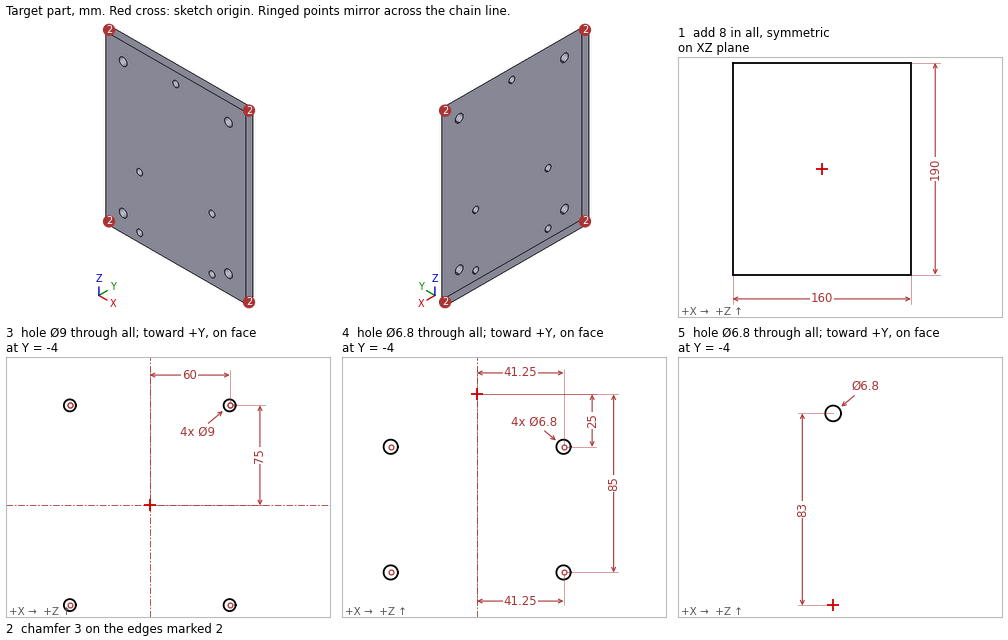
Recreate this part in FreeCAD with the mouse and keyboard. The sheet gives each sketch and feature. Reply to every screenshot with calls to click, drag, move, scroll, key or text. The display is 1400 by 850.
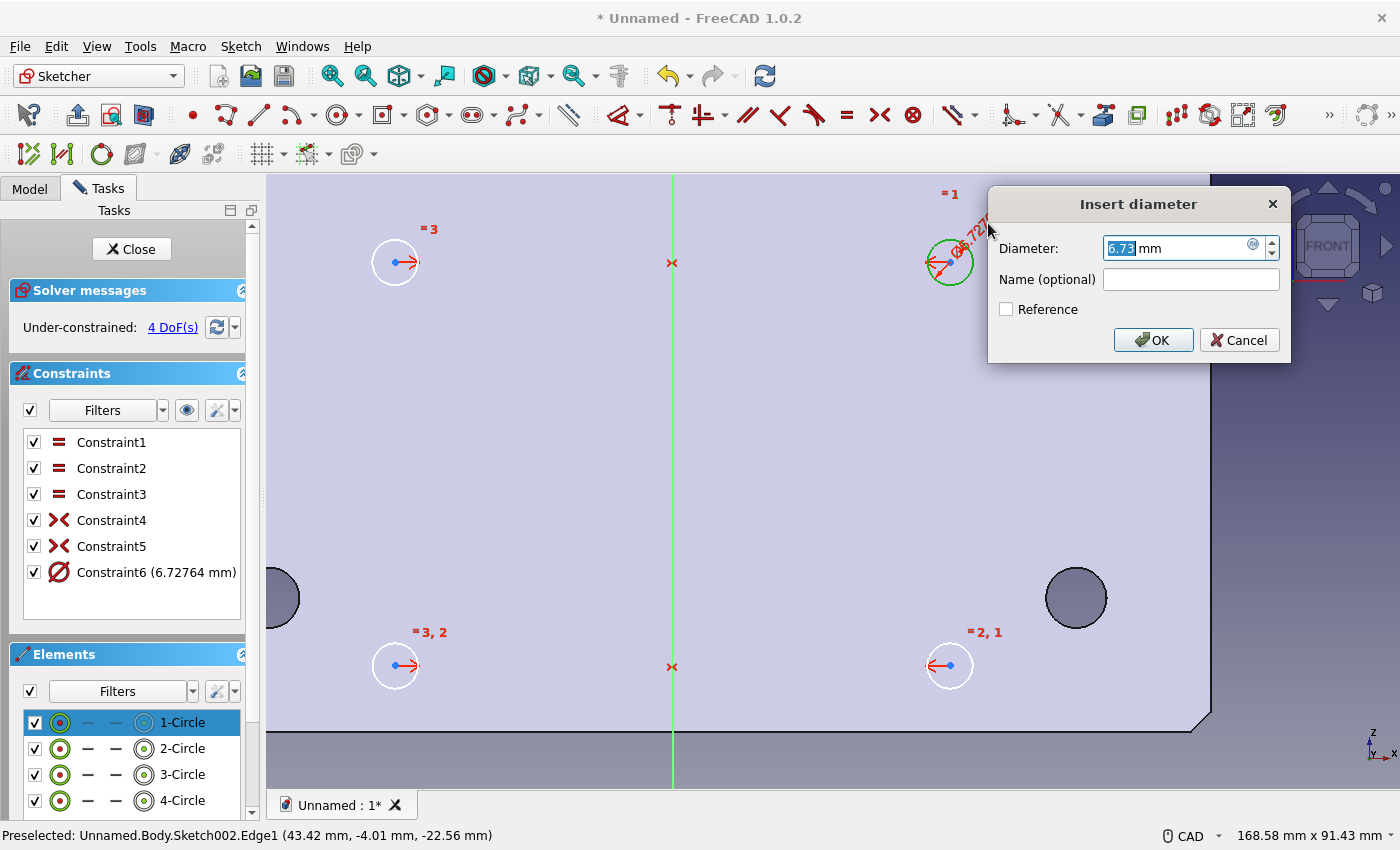
text(6.8)
key(Return)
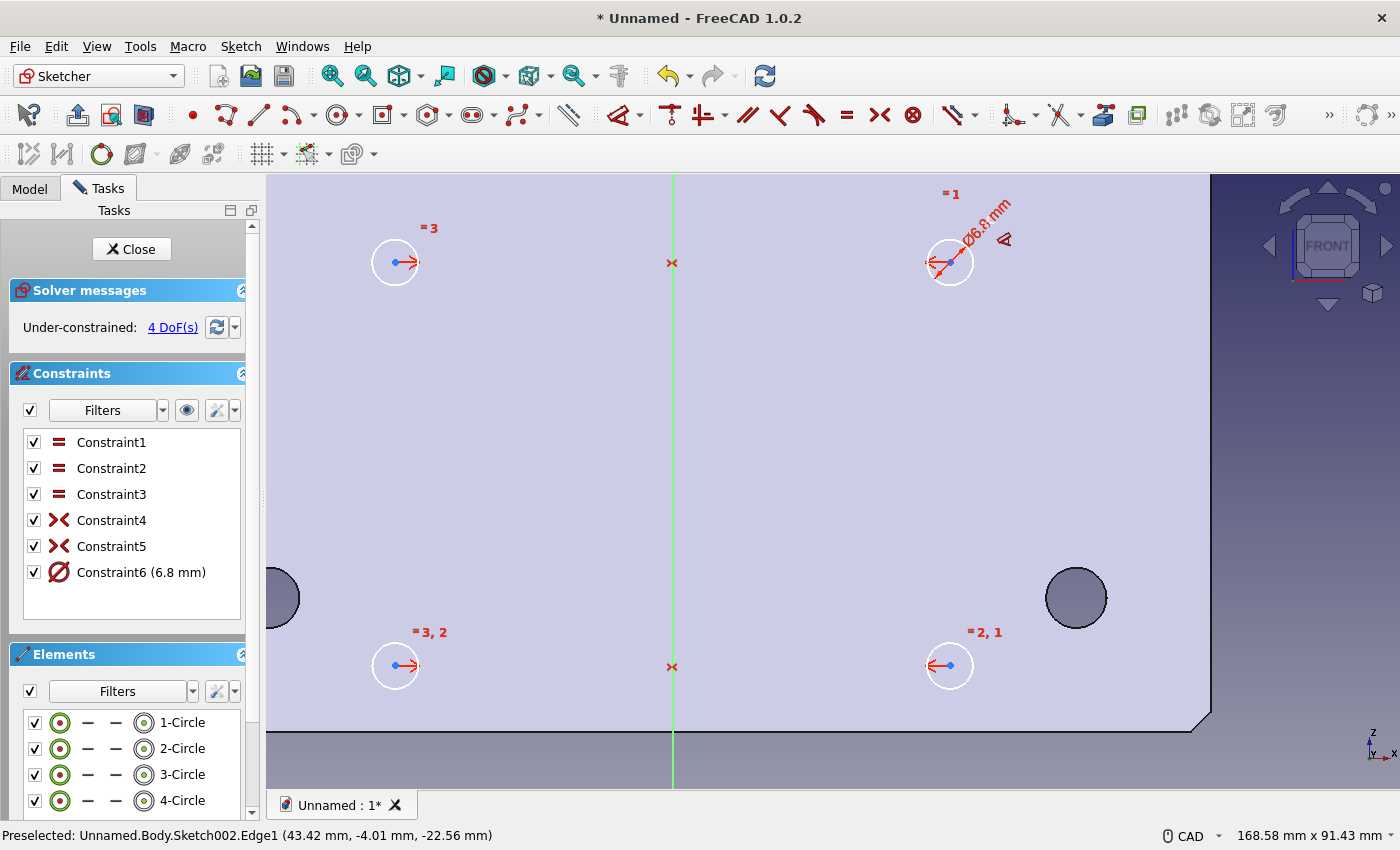
click(950, 262)
click(984, 246)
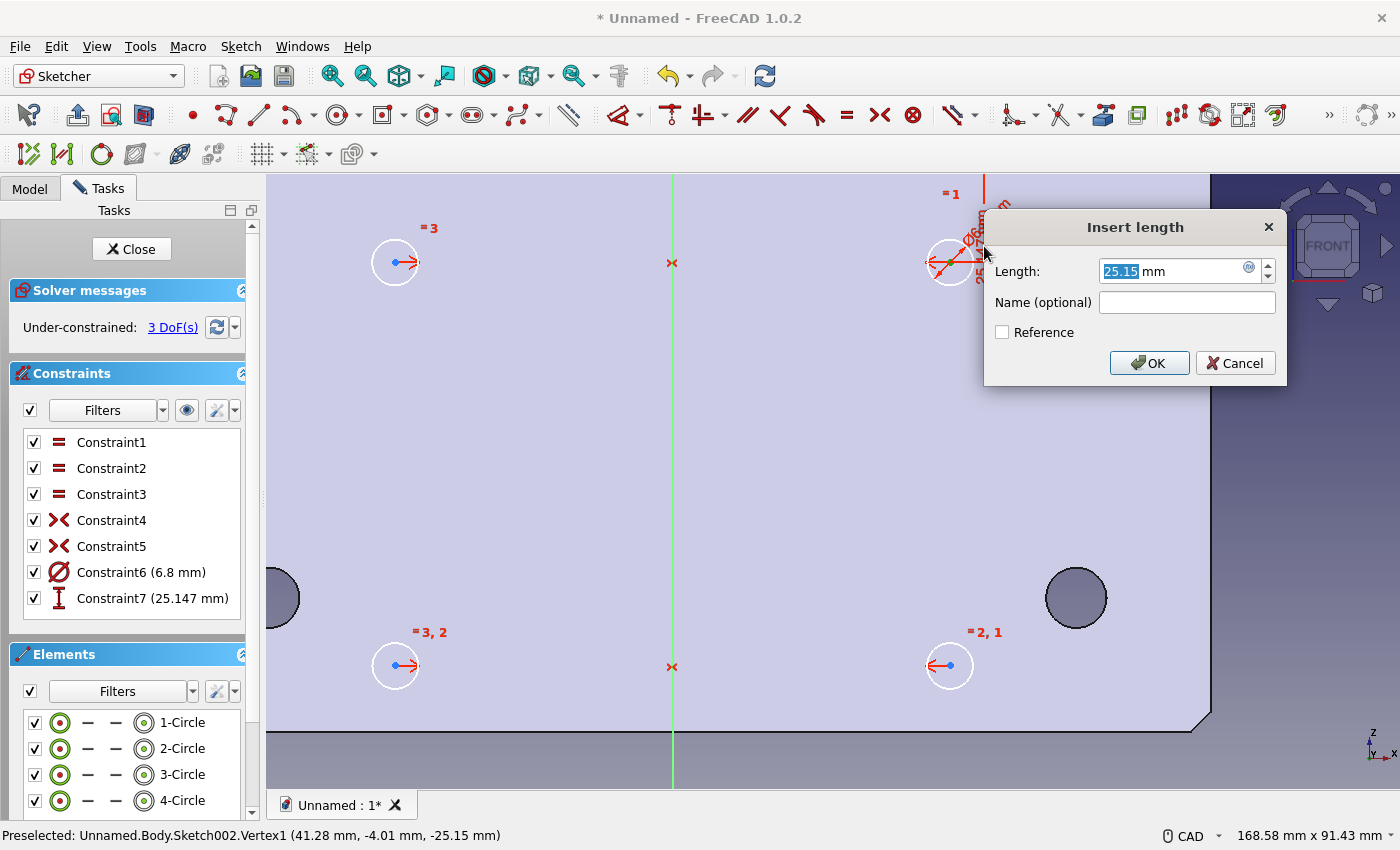
text(25)
key(Return)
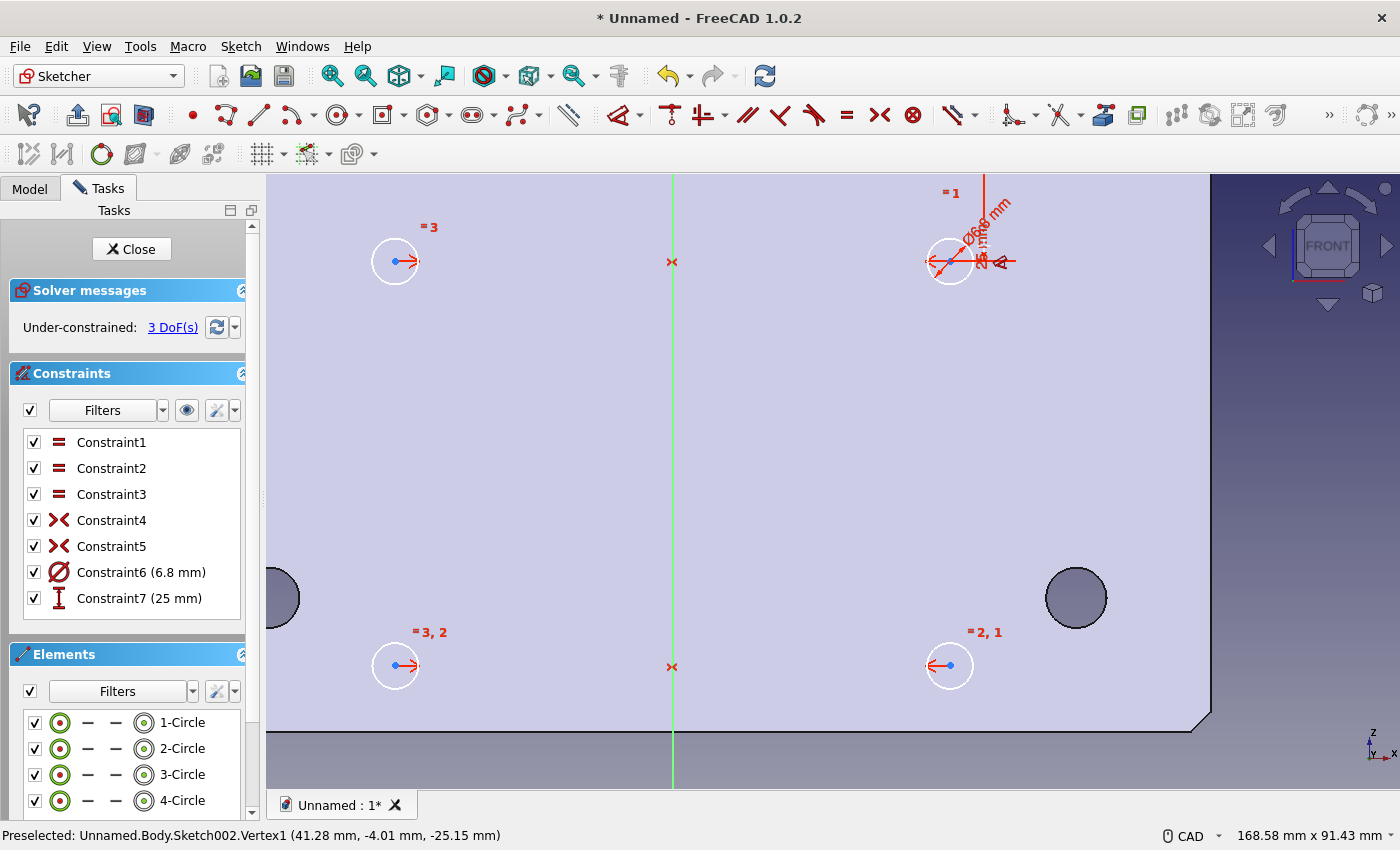
click(950, 666)
click(984, 434)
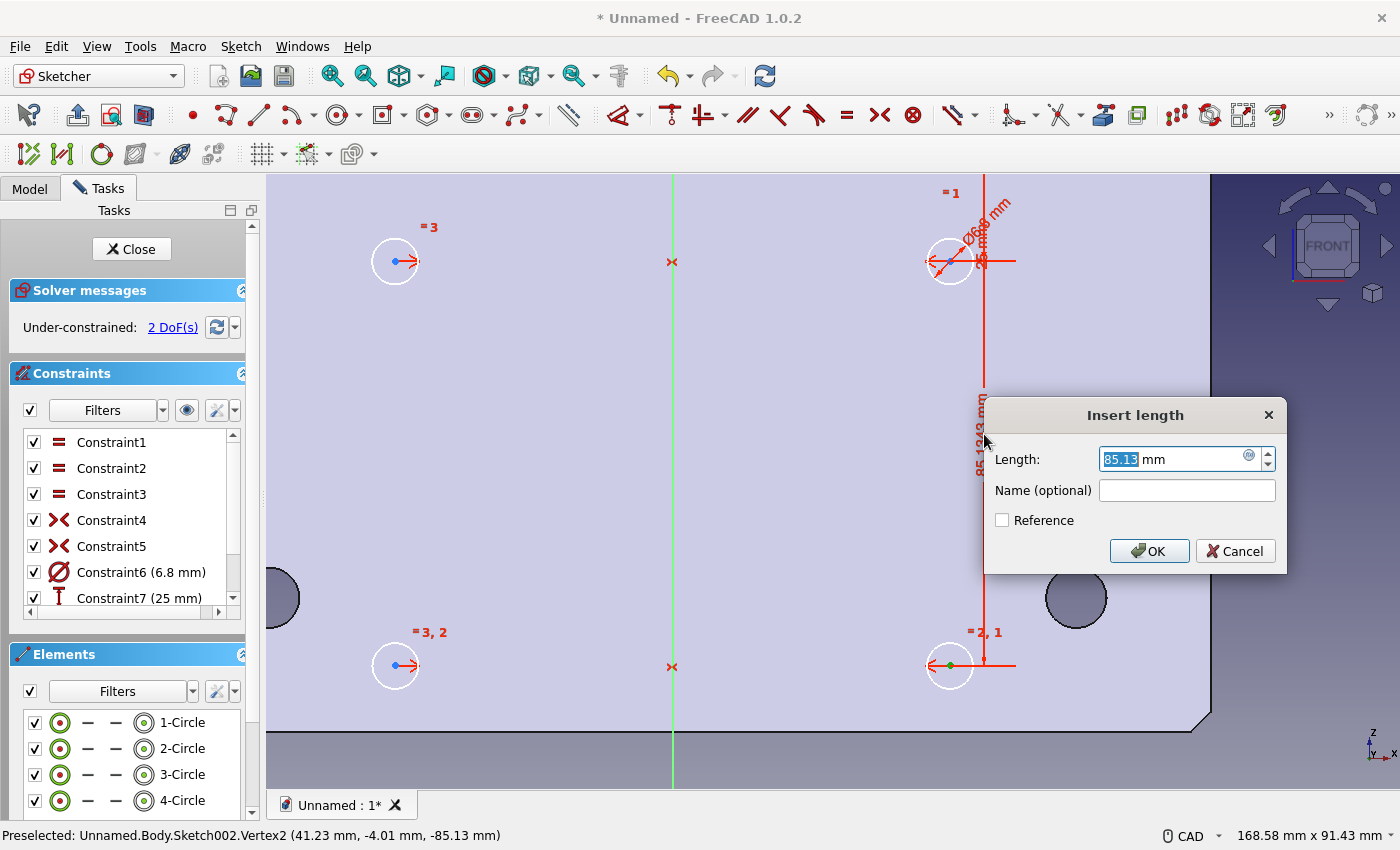
text(85)
key(Return)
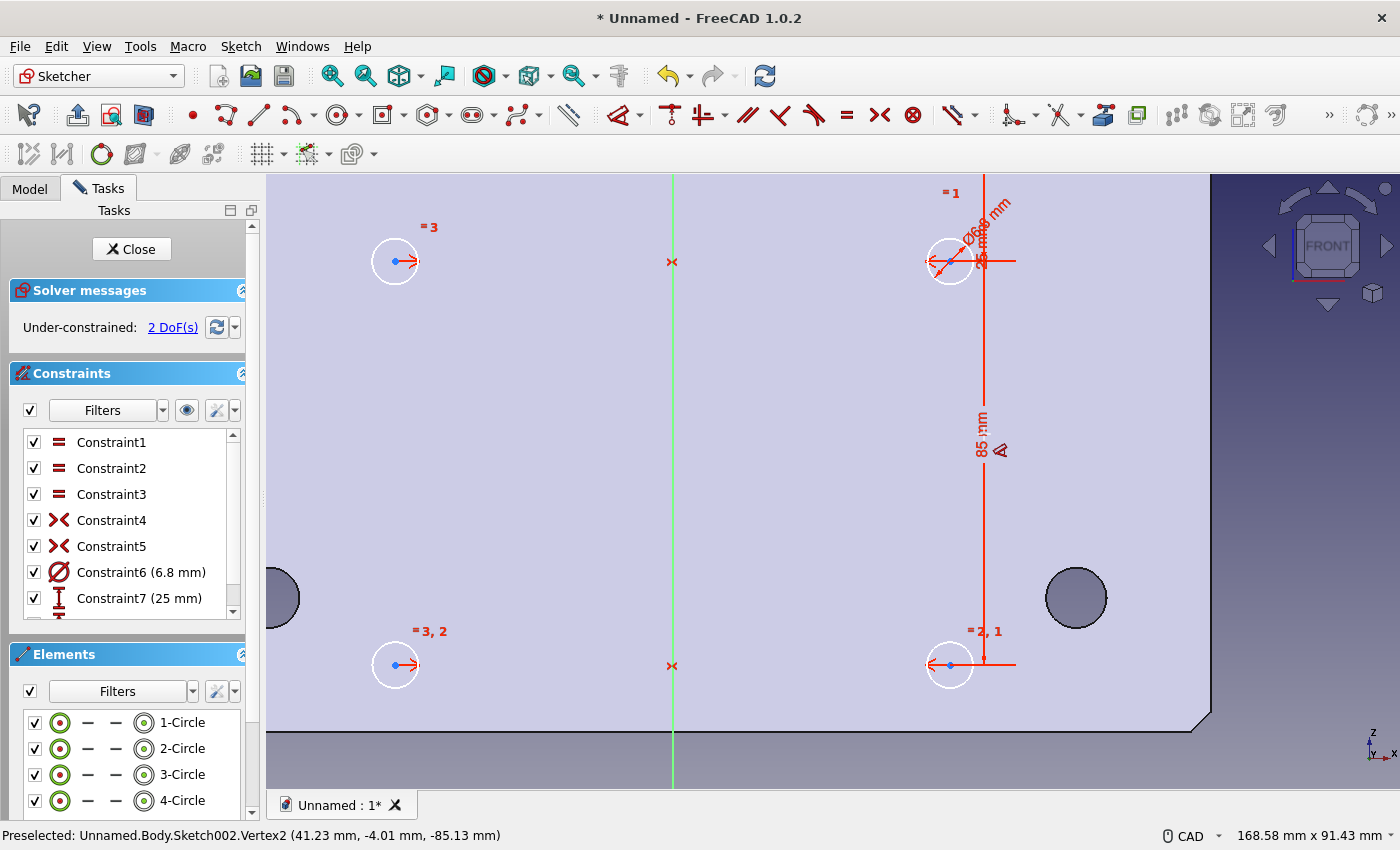
click(950, 261)
click(811, 295)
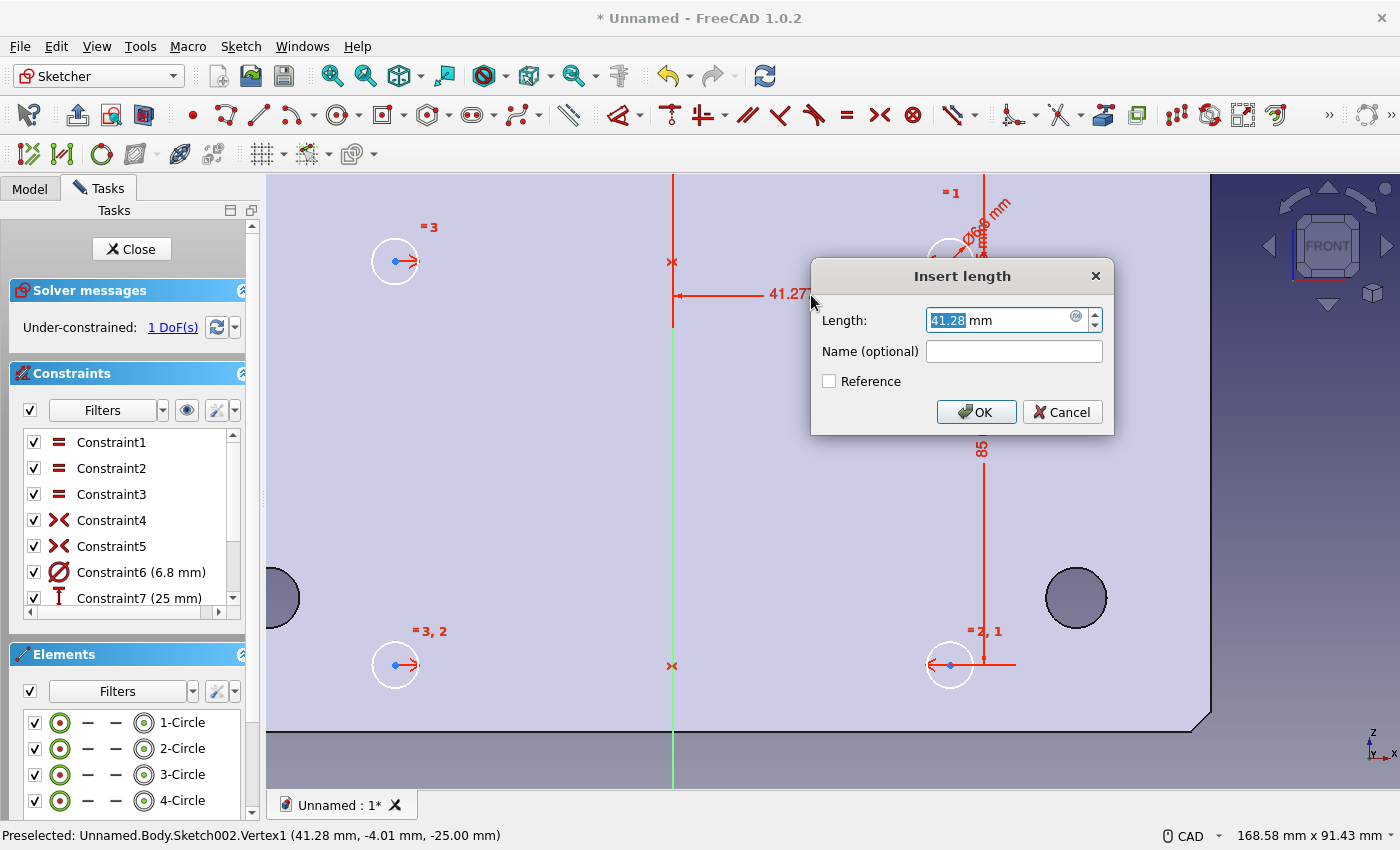
text(41.25)
key(Return)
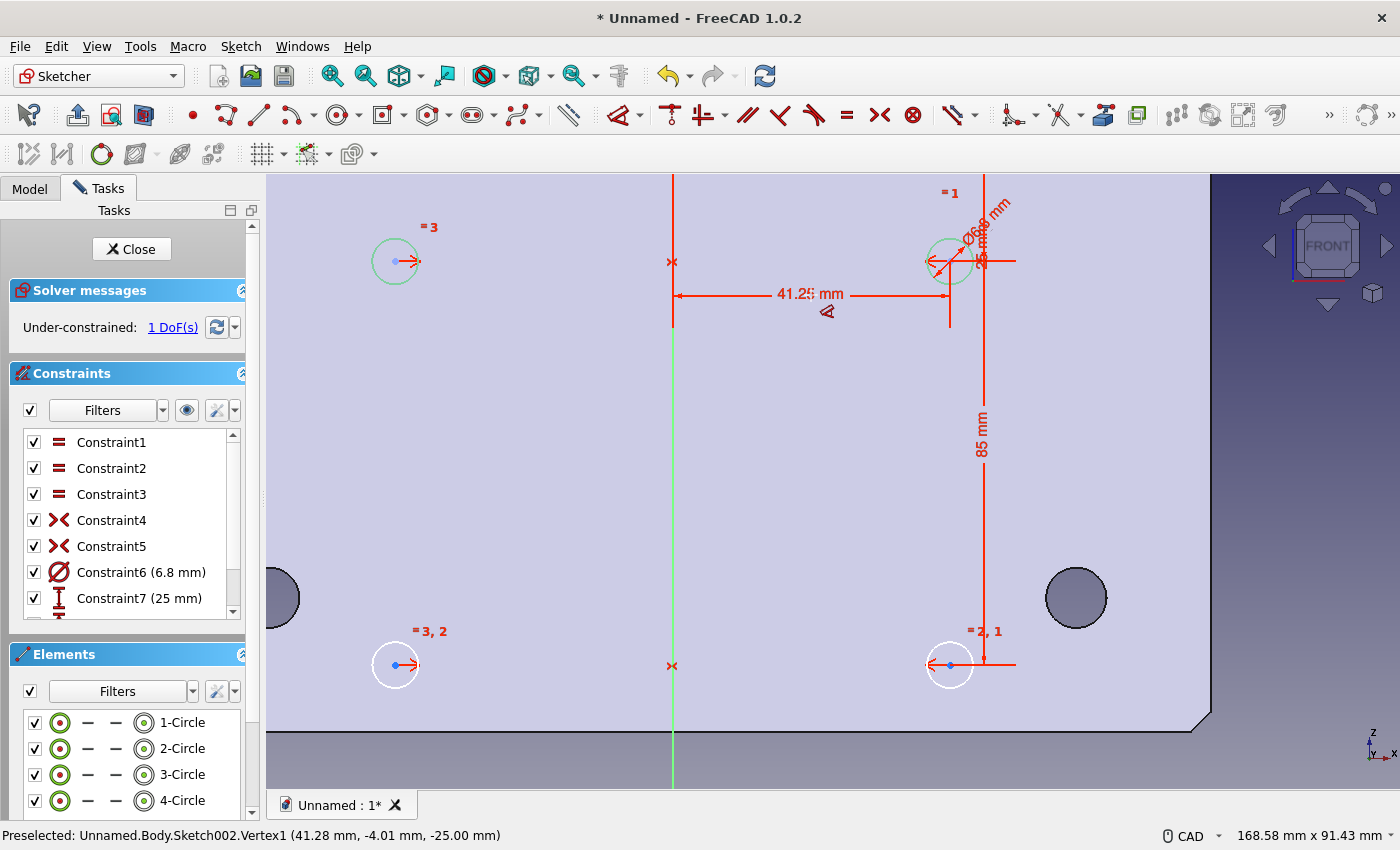
click(950, 665)
click(811, 699)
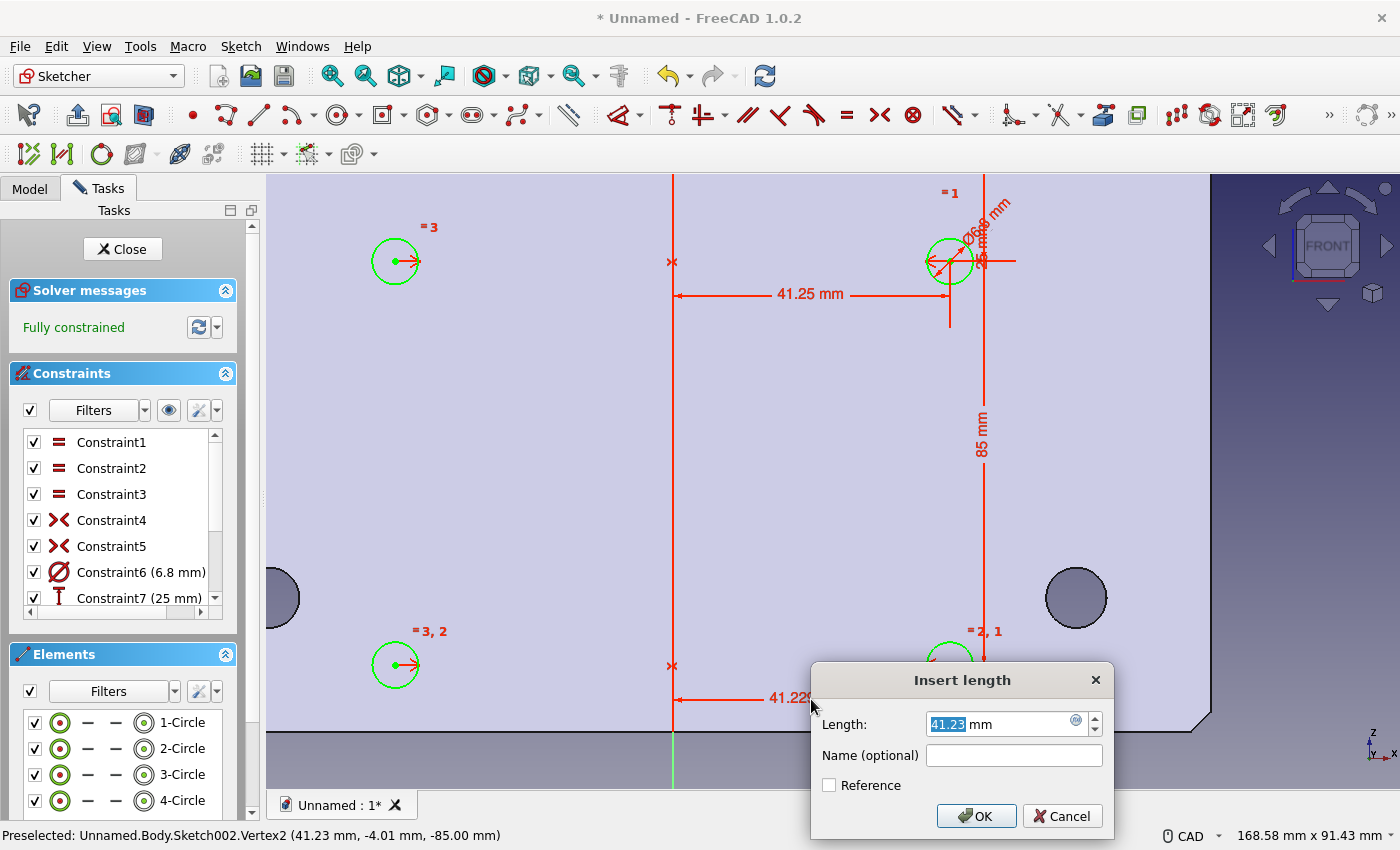
text(41.25)
key(Return)
key(Escape)